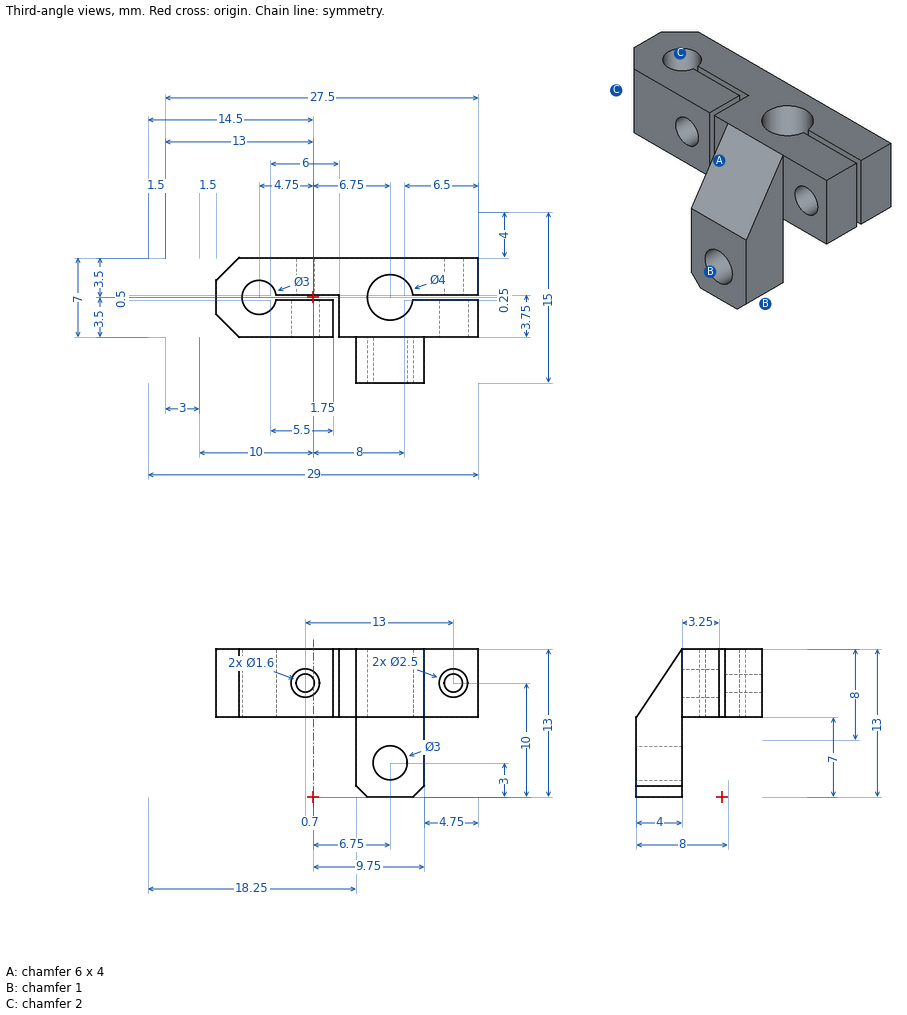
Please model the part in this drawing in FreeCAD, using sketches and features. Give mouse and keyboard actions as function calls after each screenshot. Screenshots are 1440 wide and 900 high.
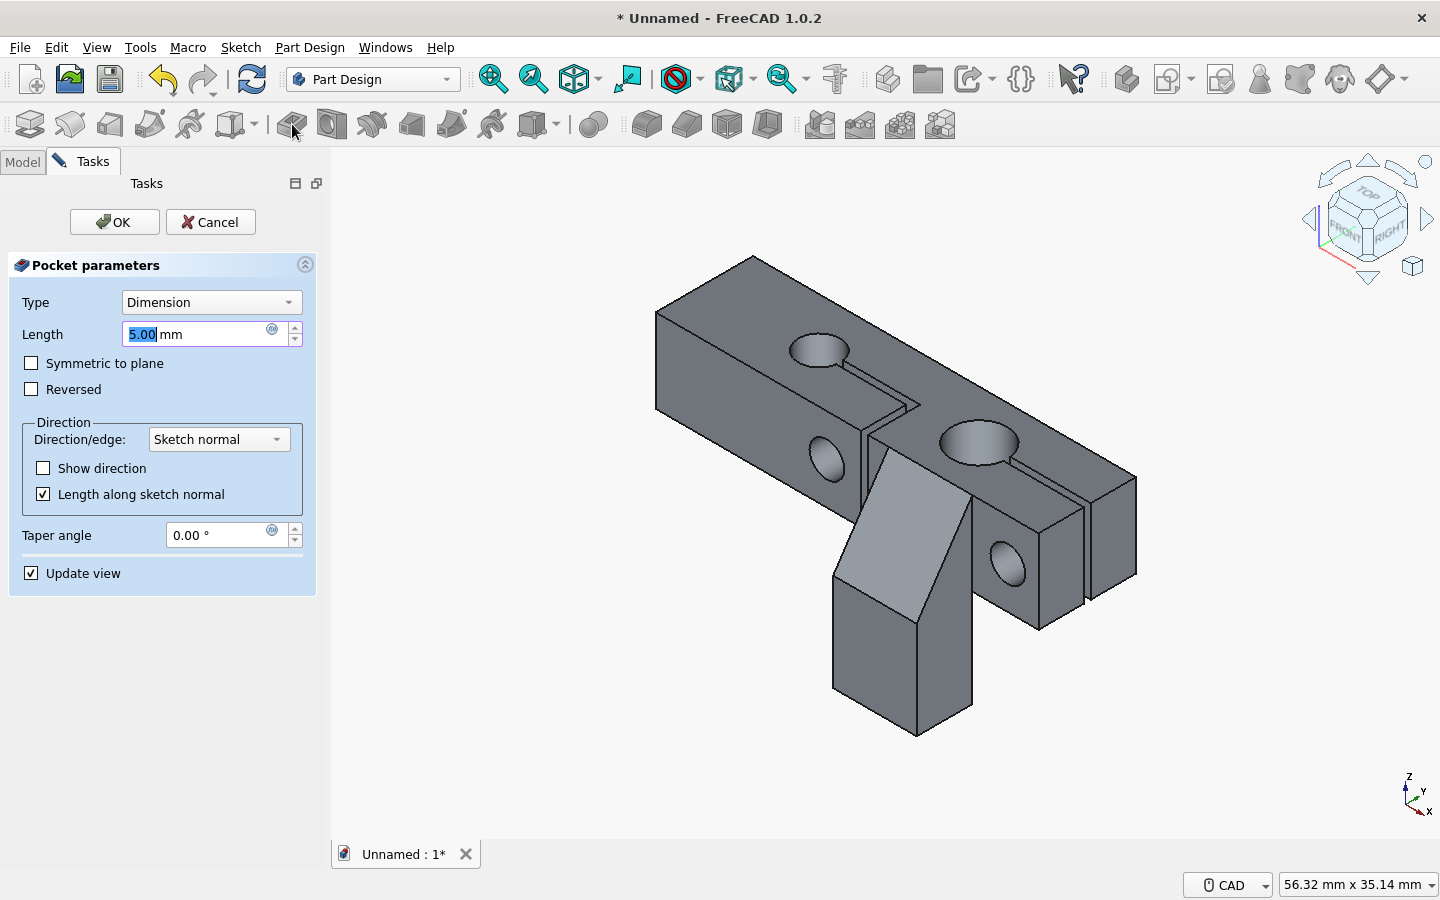
text(3.25)
key(Tab)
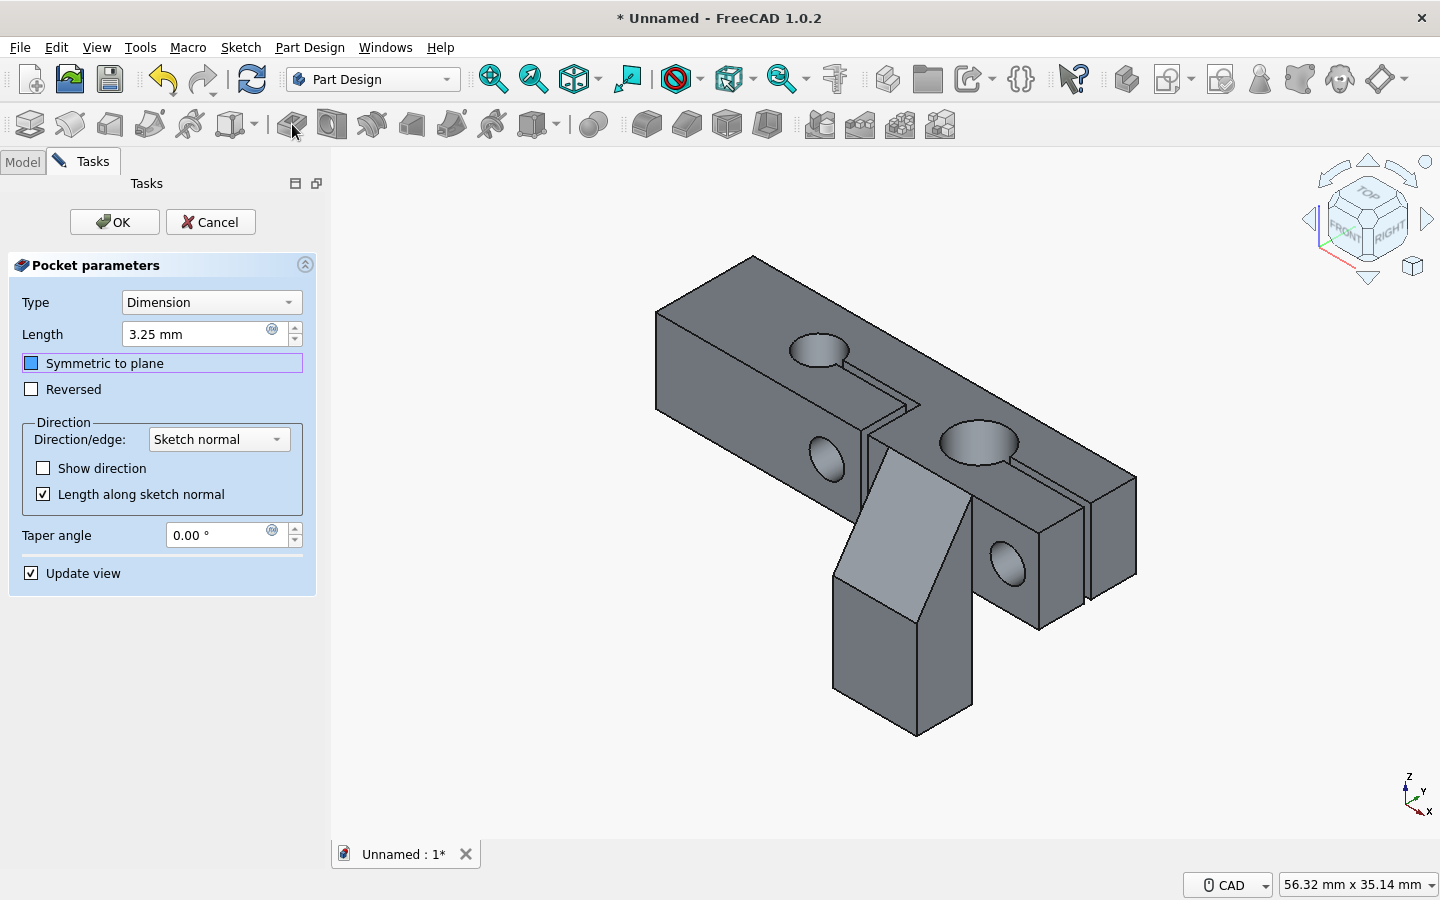
click(115, 222)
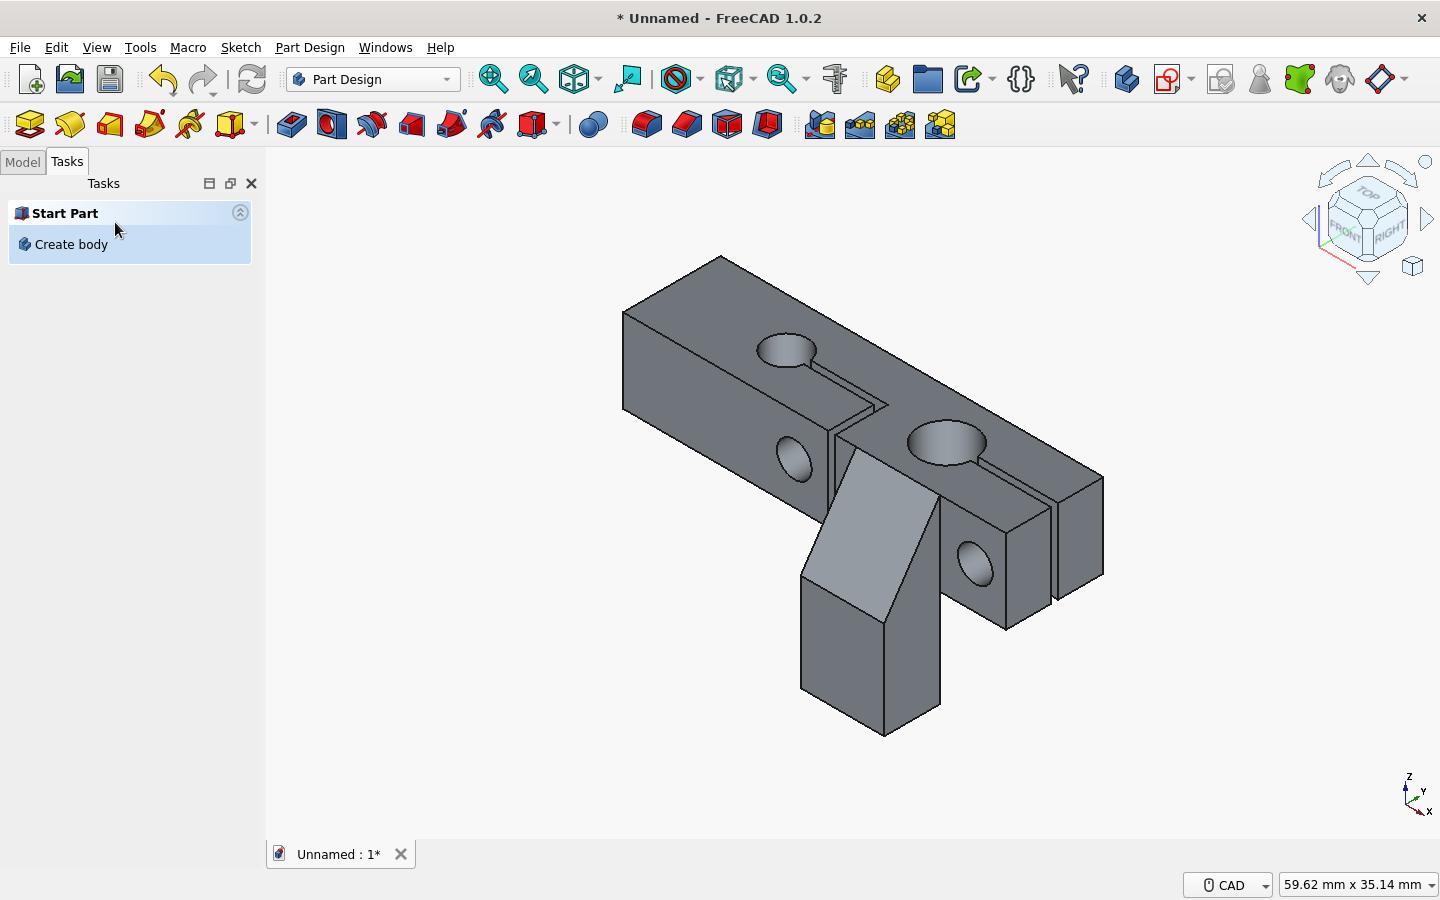
click(713, 291)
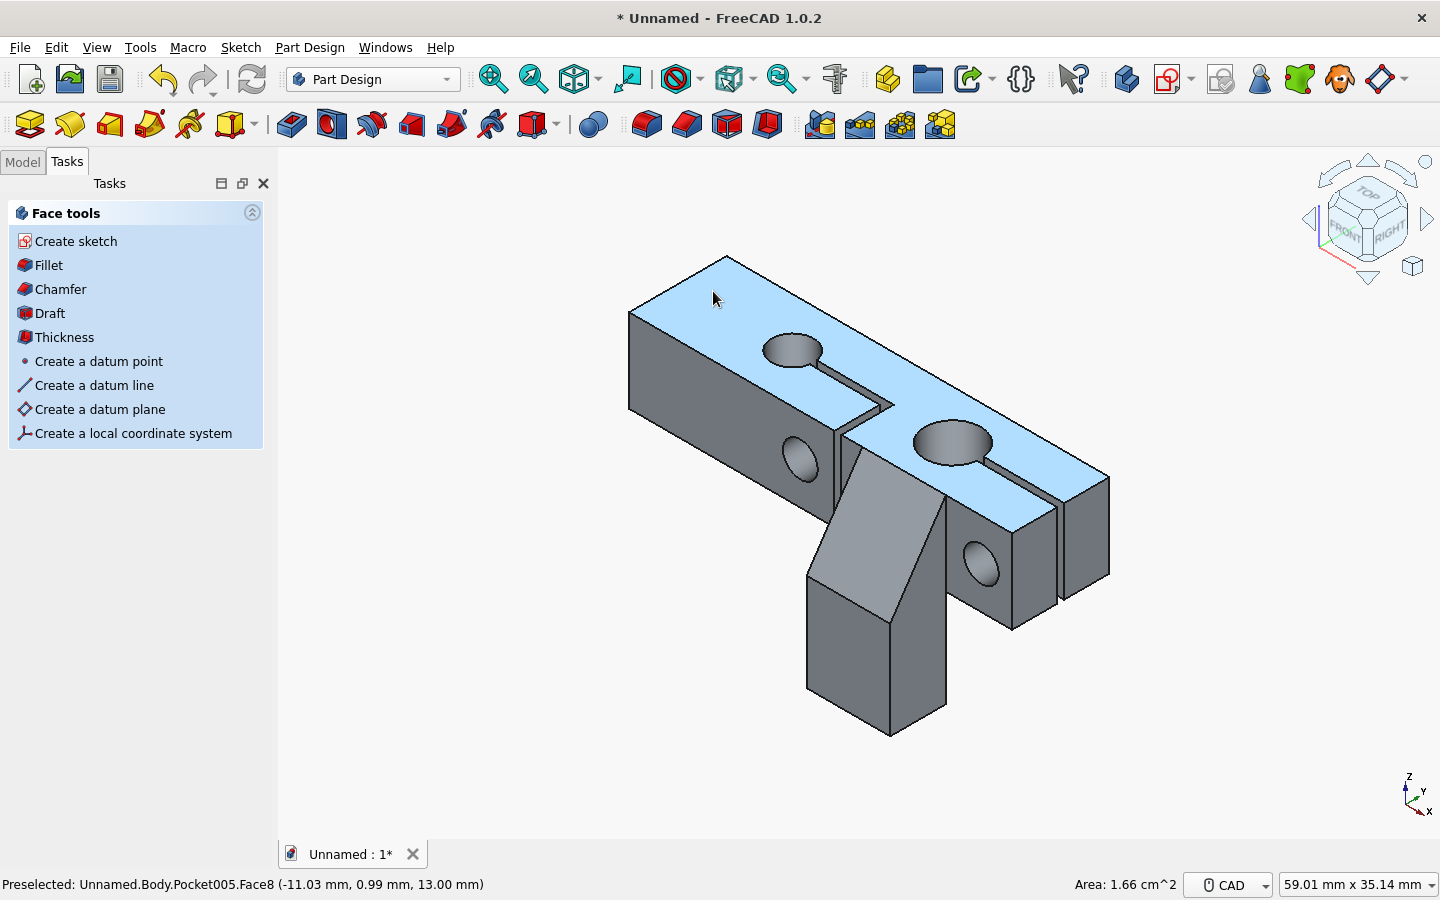
click(1168, 80)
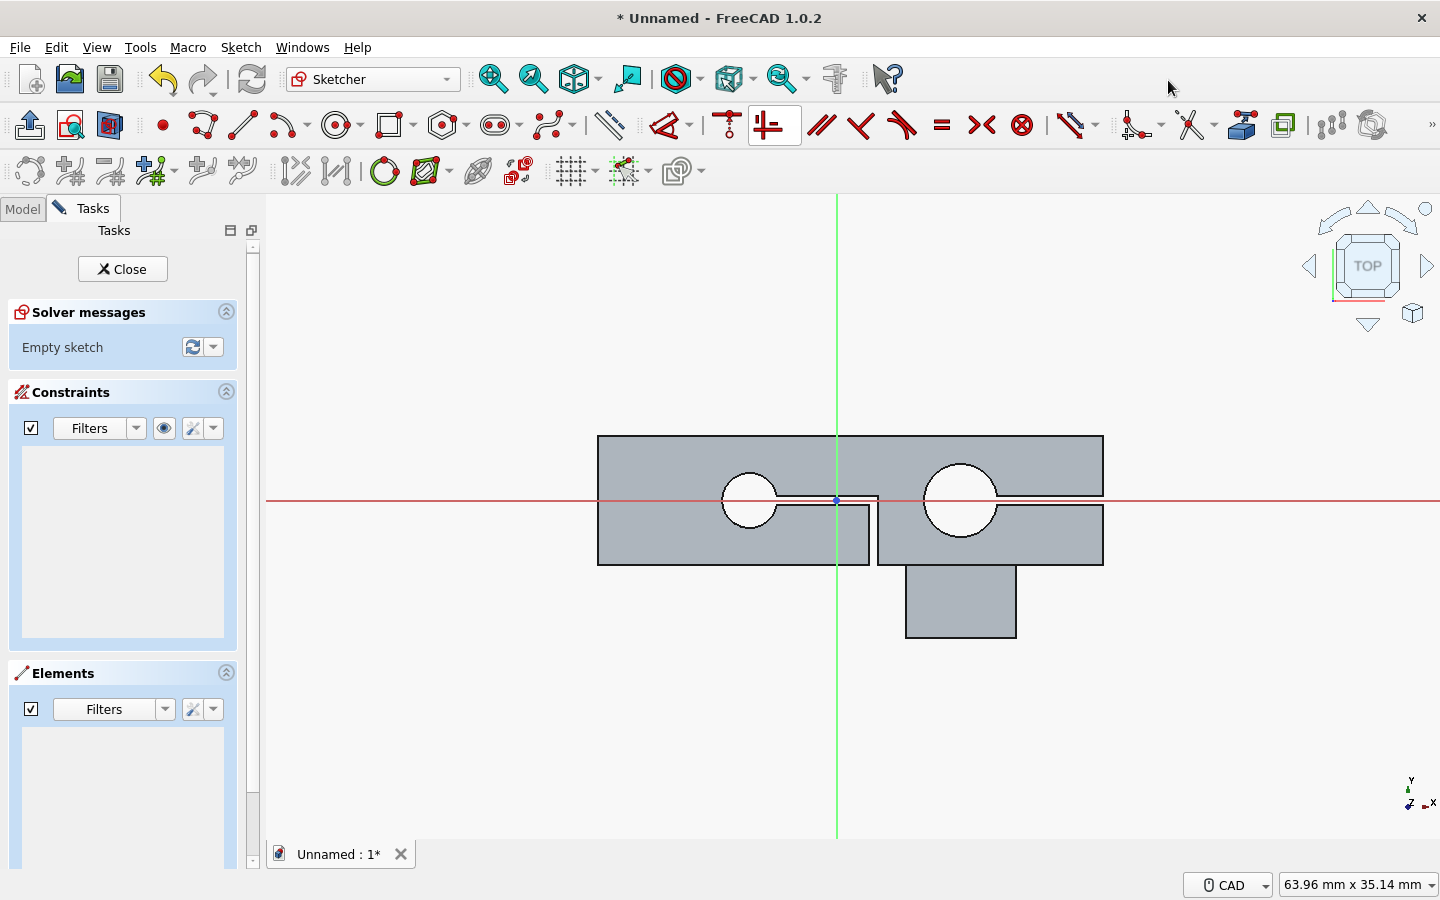
scroll(679, 491, up, 5)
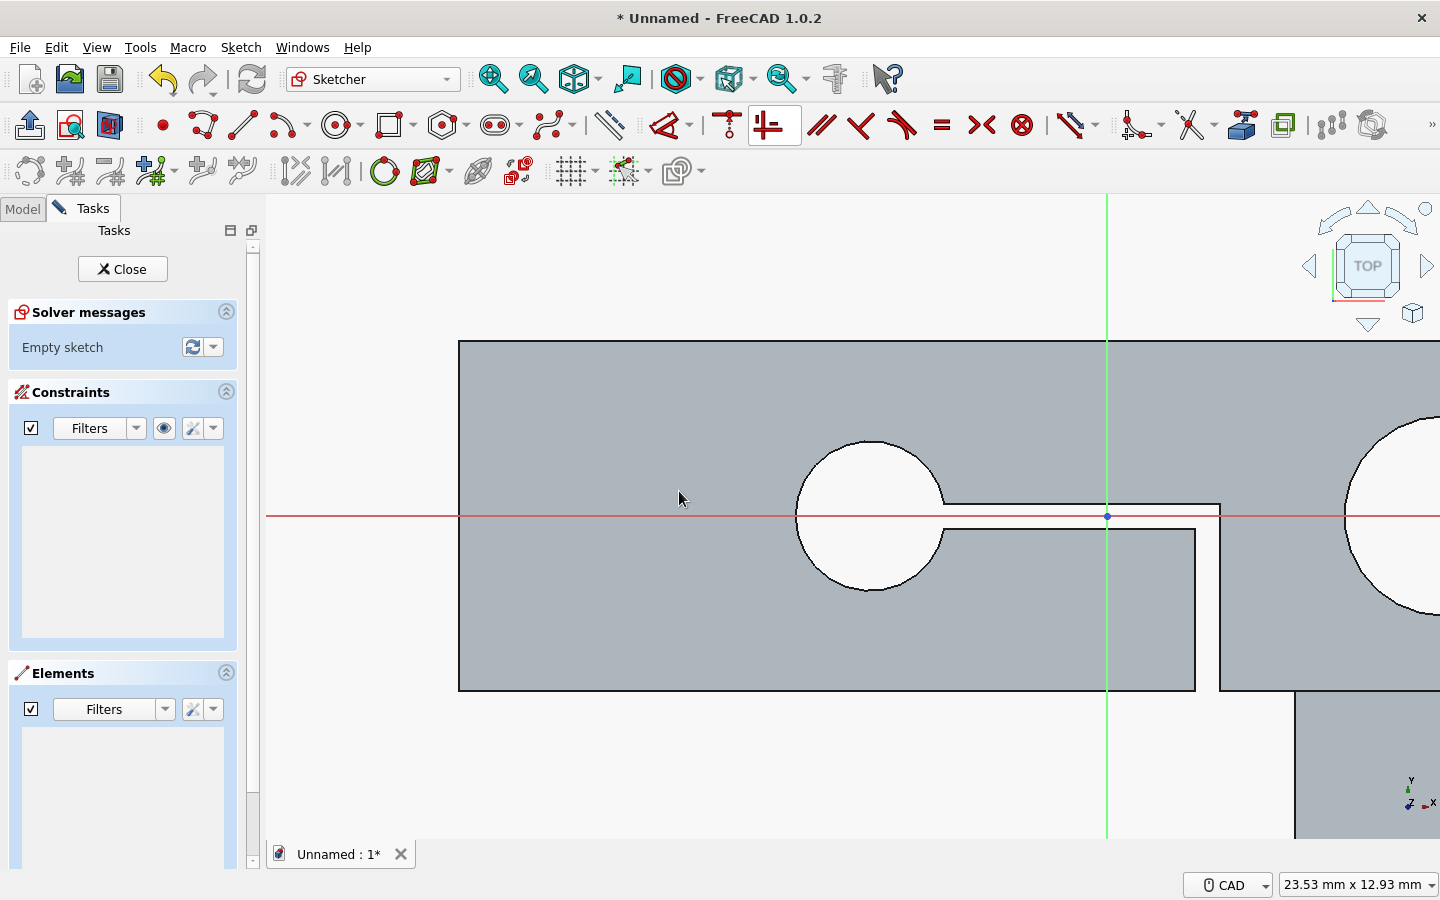
click(390, 126)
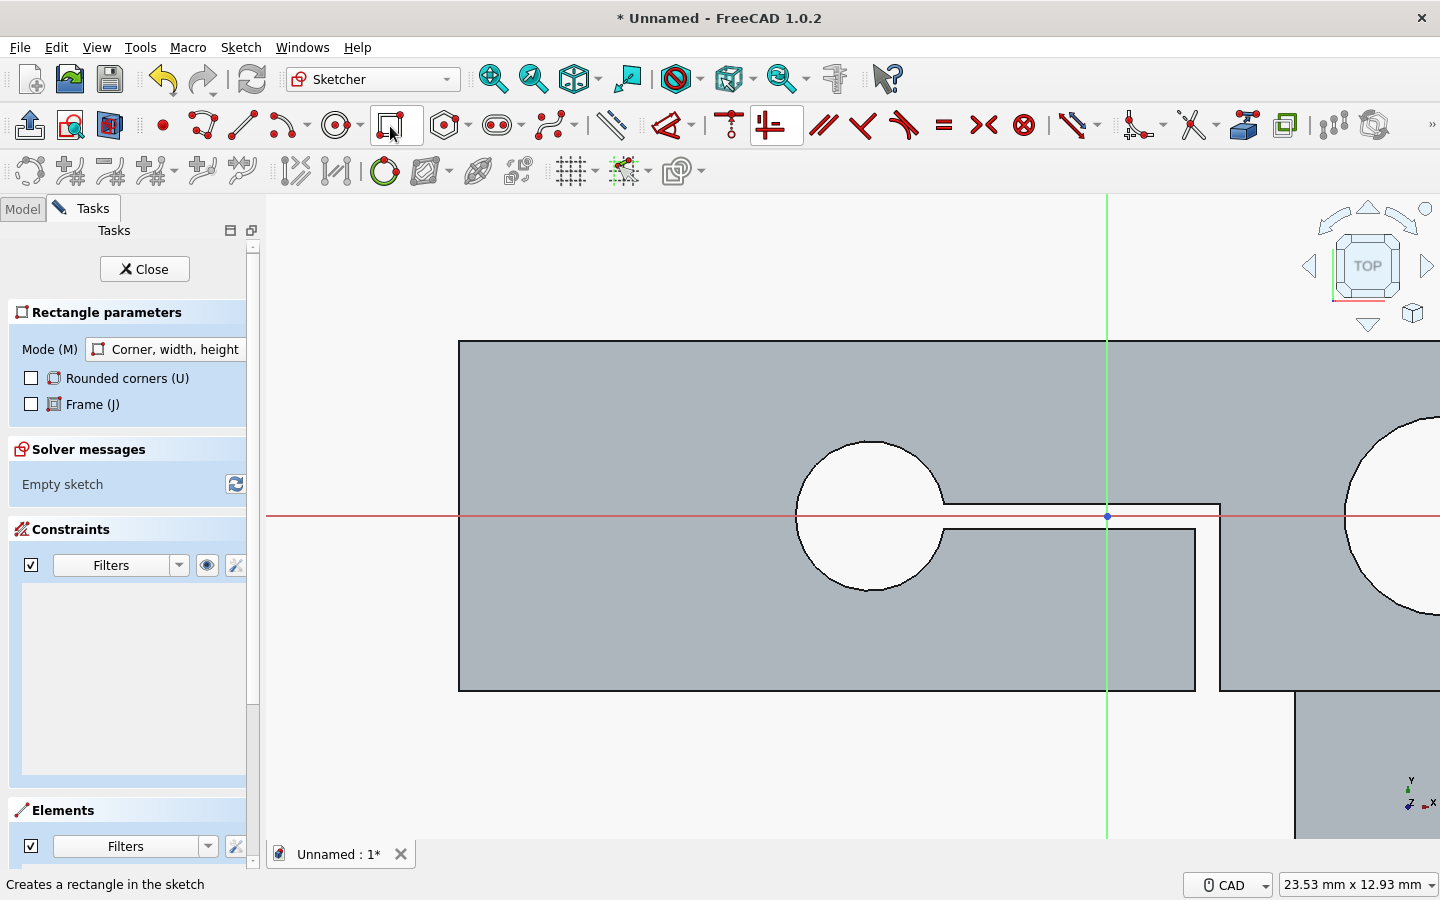
click(459, 341)
move(609, 691)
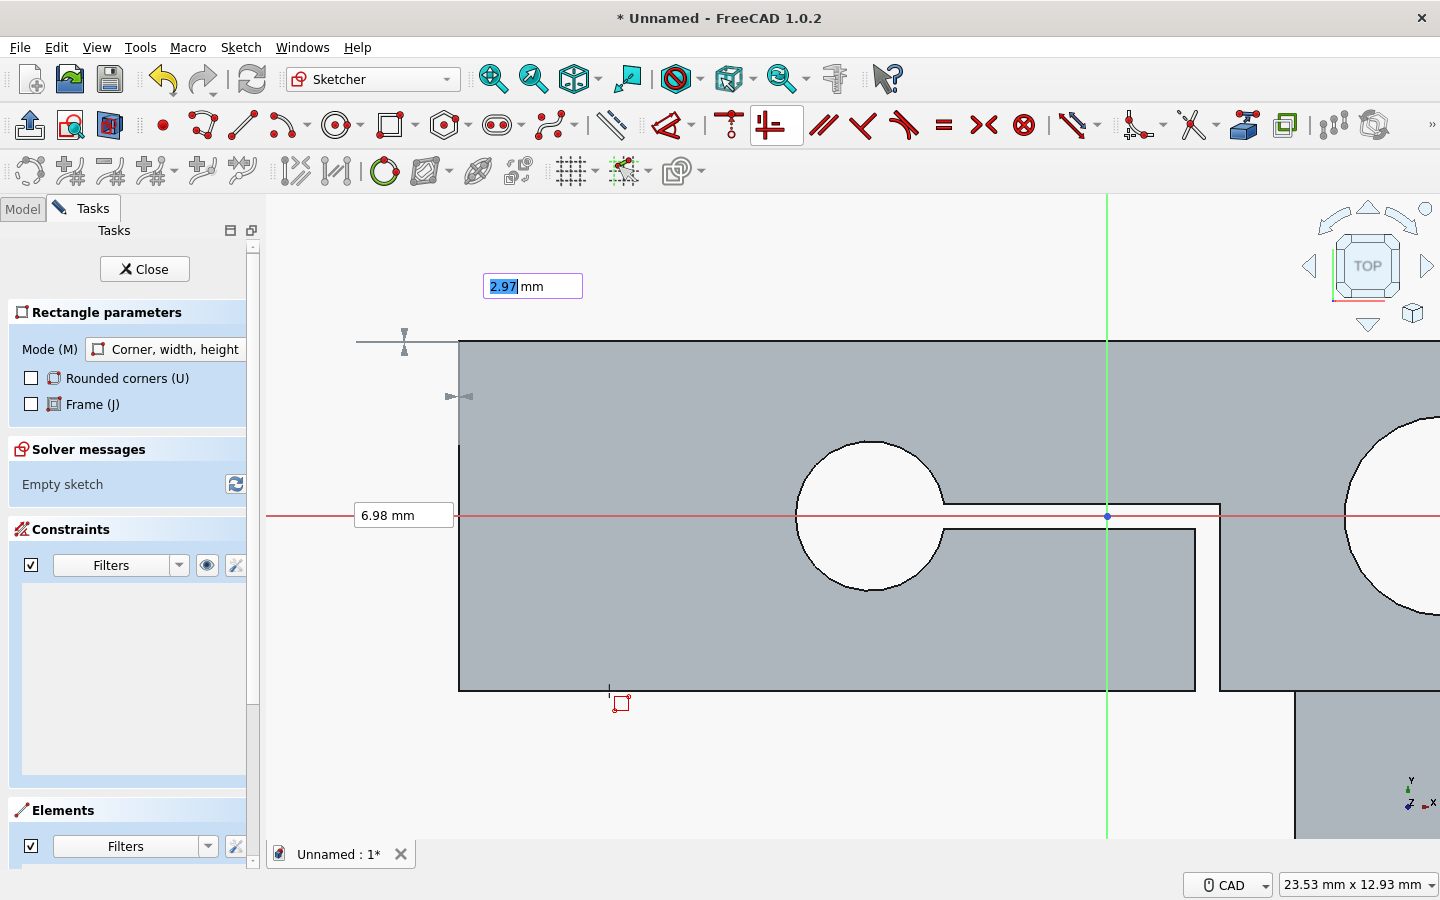
text(3)
key(Tab)
text(7)
key(Return)
key(Escape)